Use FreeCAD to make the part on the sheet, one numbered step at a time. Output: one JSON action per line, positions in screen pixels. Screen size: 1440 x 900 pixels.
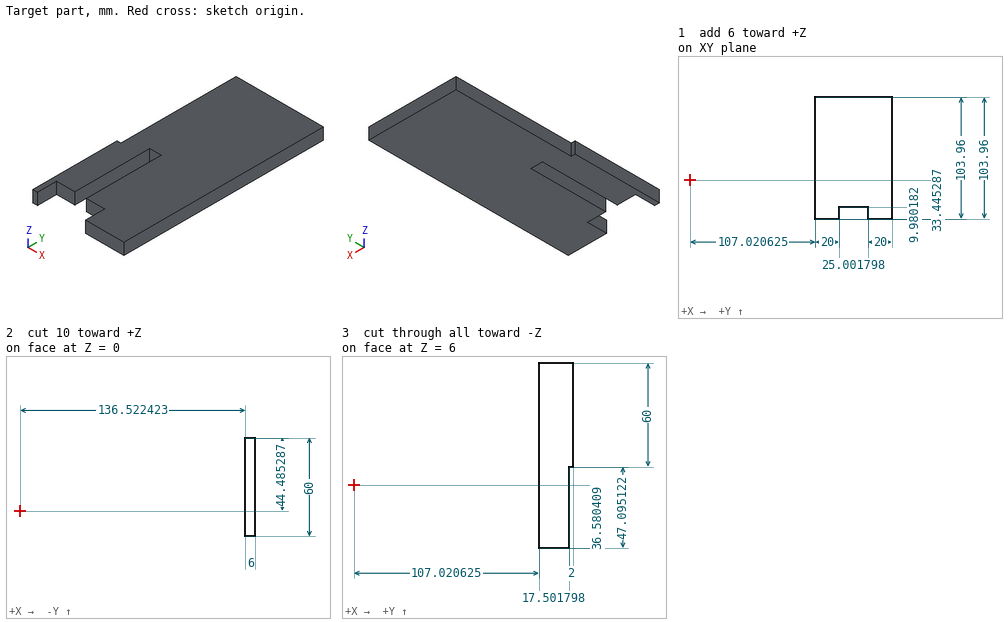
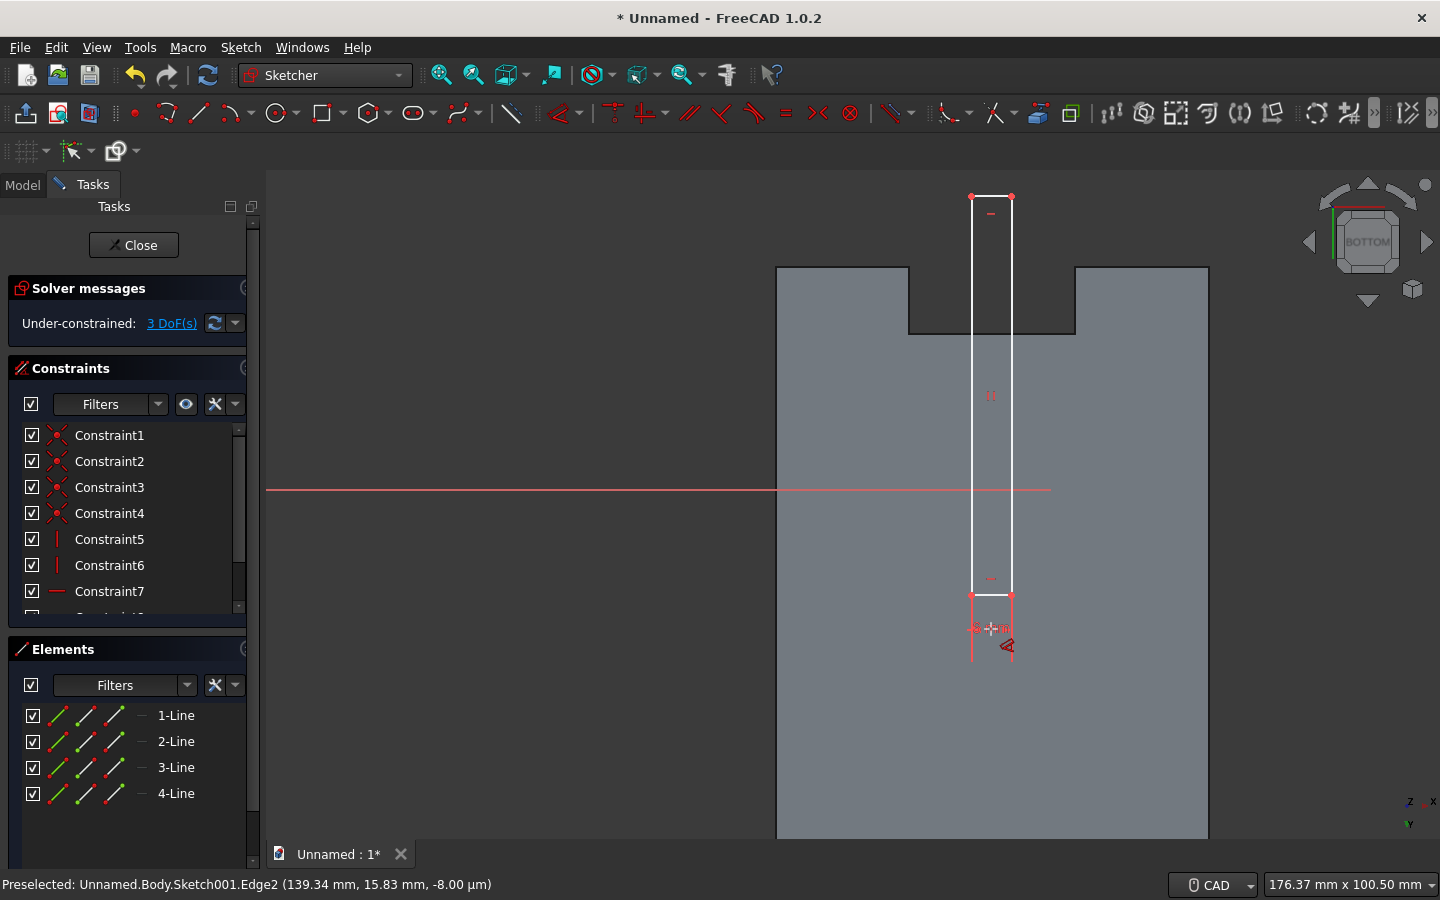
{"action": "left_click", "coordinate": [972, 316]}
{"action": "left_click", "coordinate": [938, 397]}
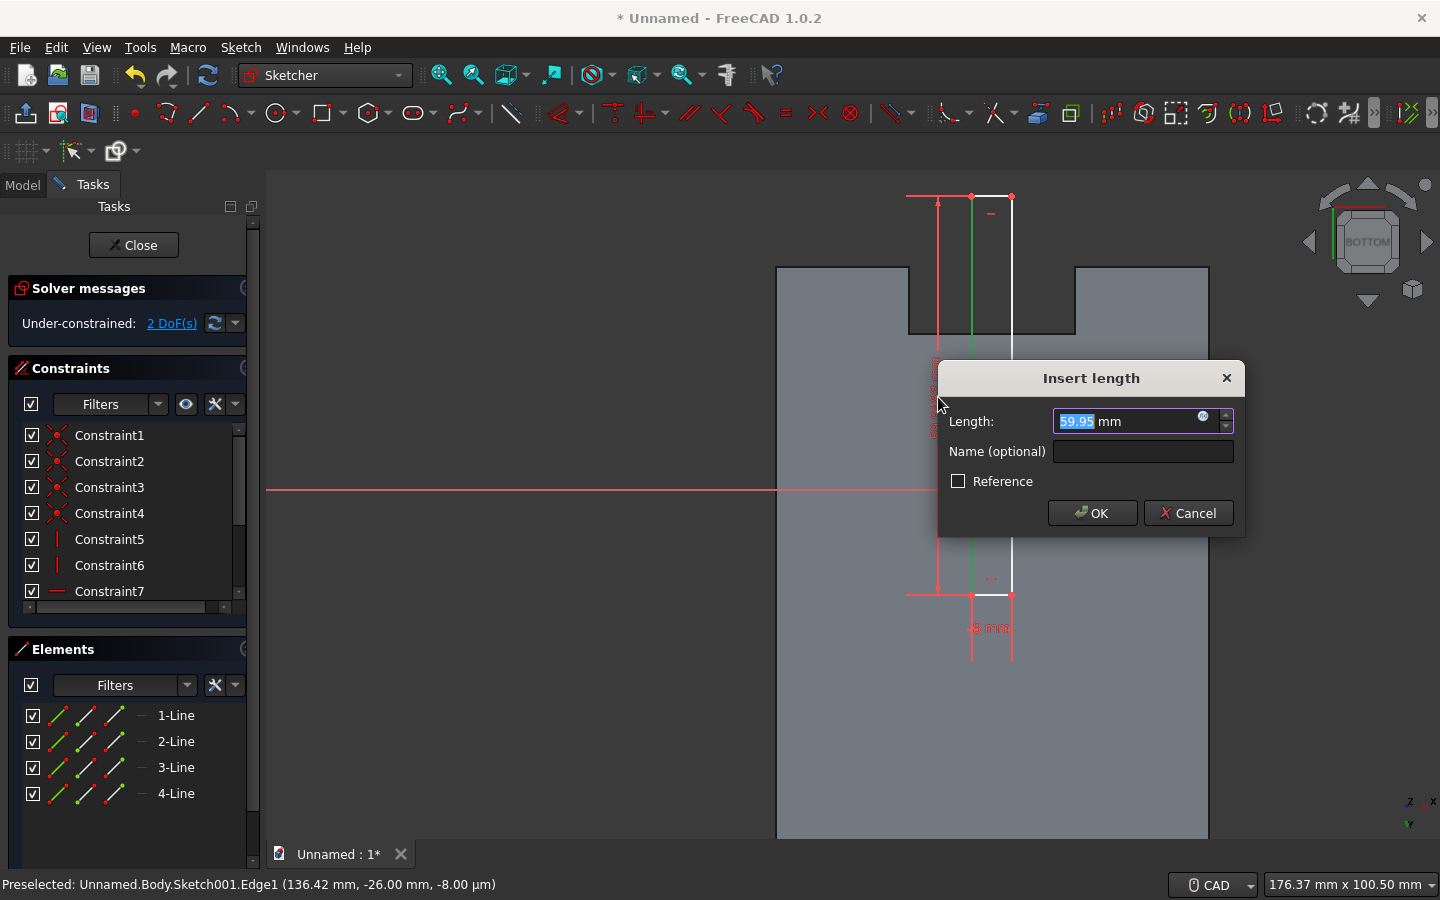
{"action": "type", "text": "60"}
{"action": "key", "text": "Return"}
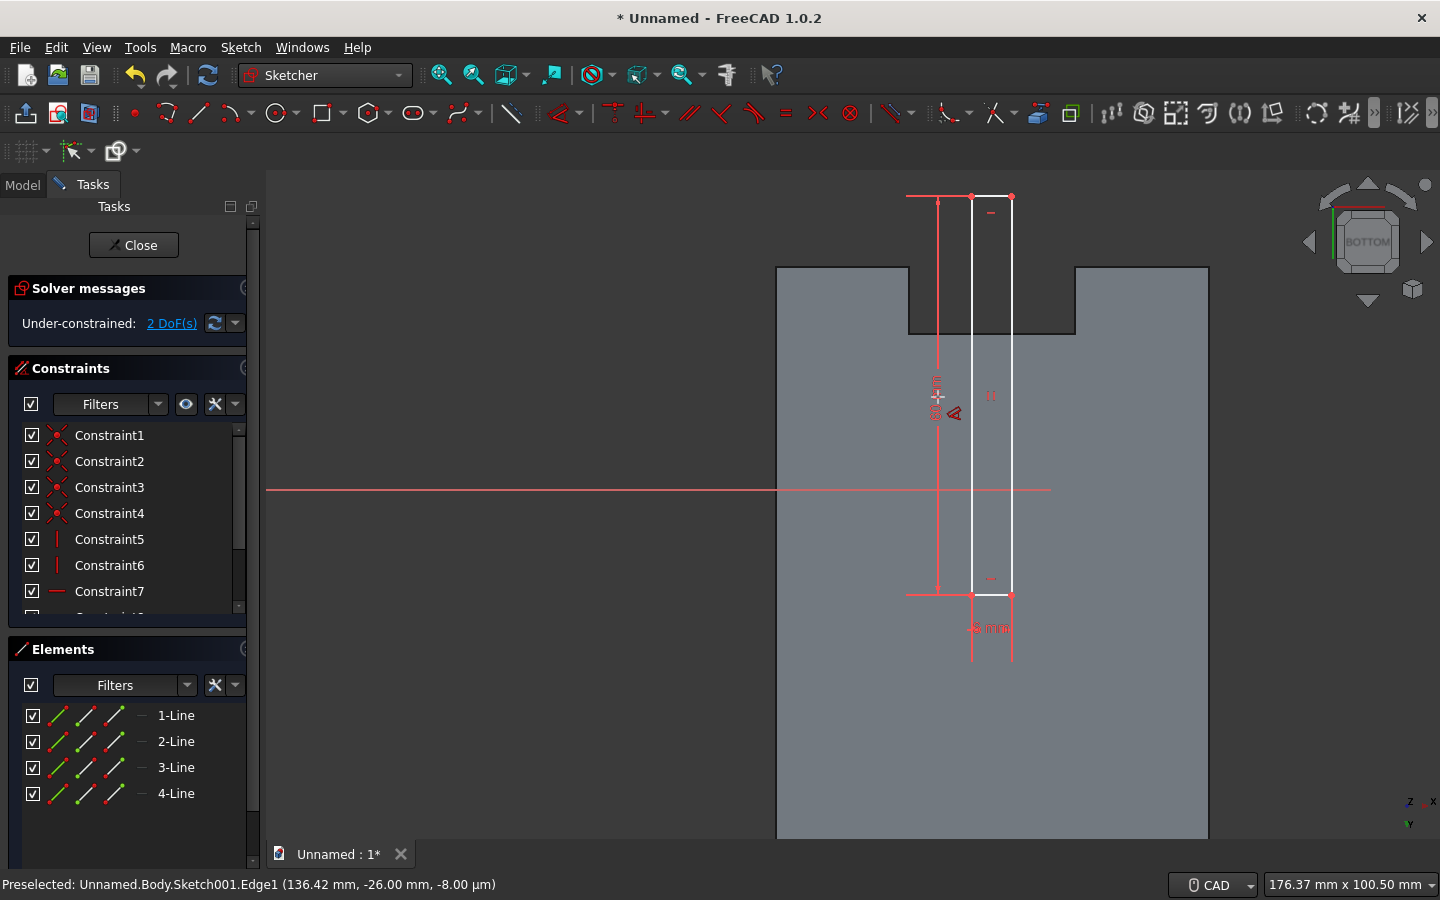
{"action": "scroll", "coordinate": [1275, 730], "scroll_direction": "down", "scroll_amount": 2}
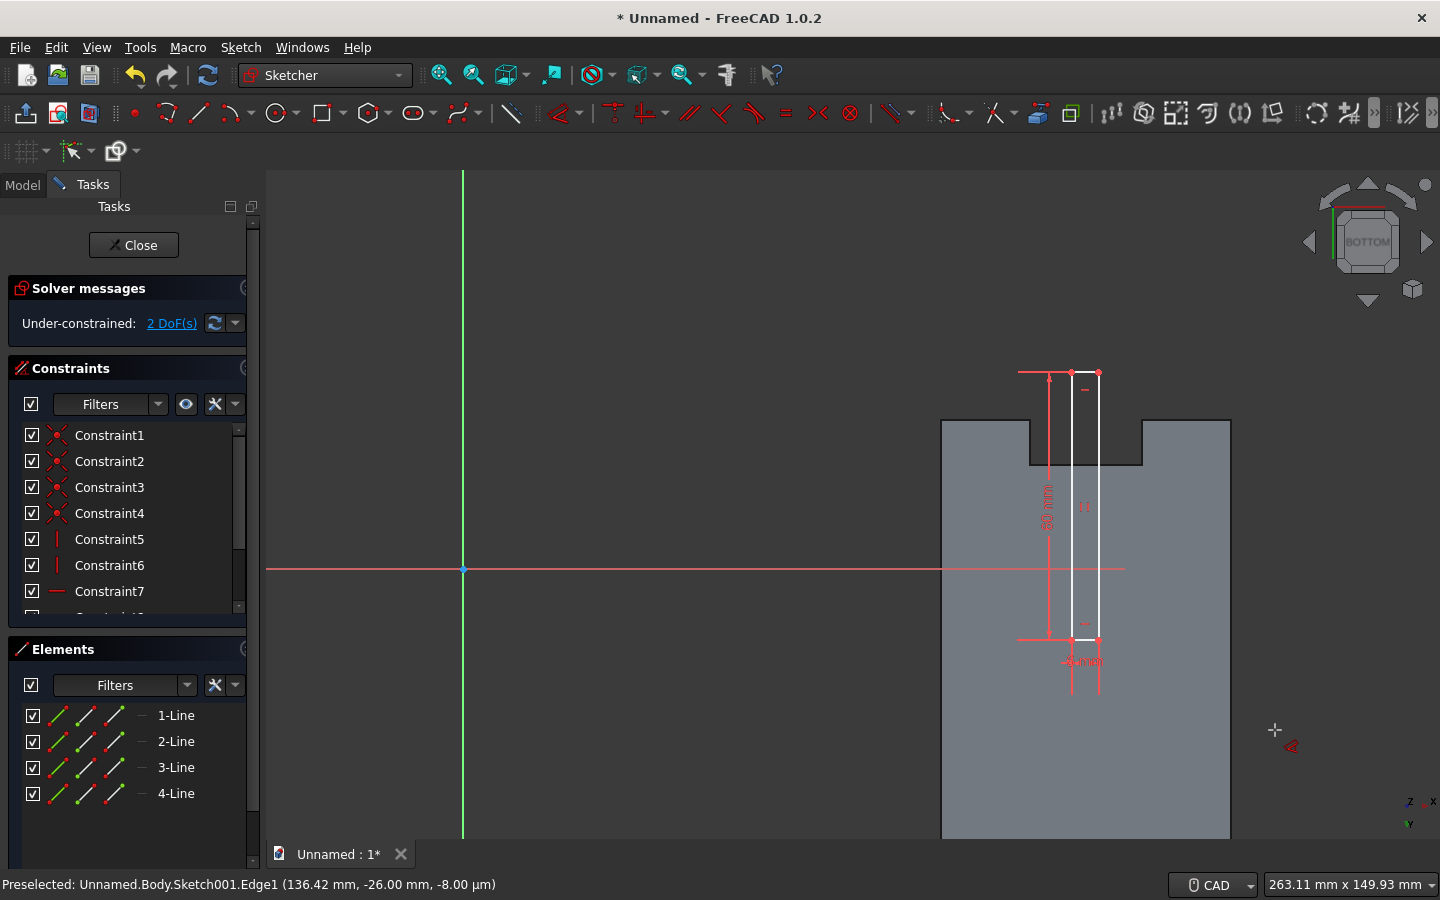
{"action": "left_click", "coordinate": [1072, 372]}
{"action": "left_click", "coordinate": [429, 471]}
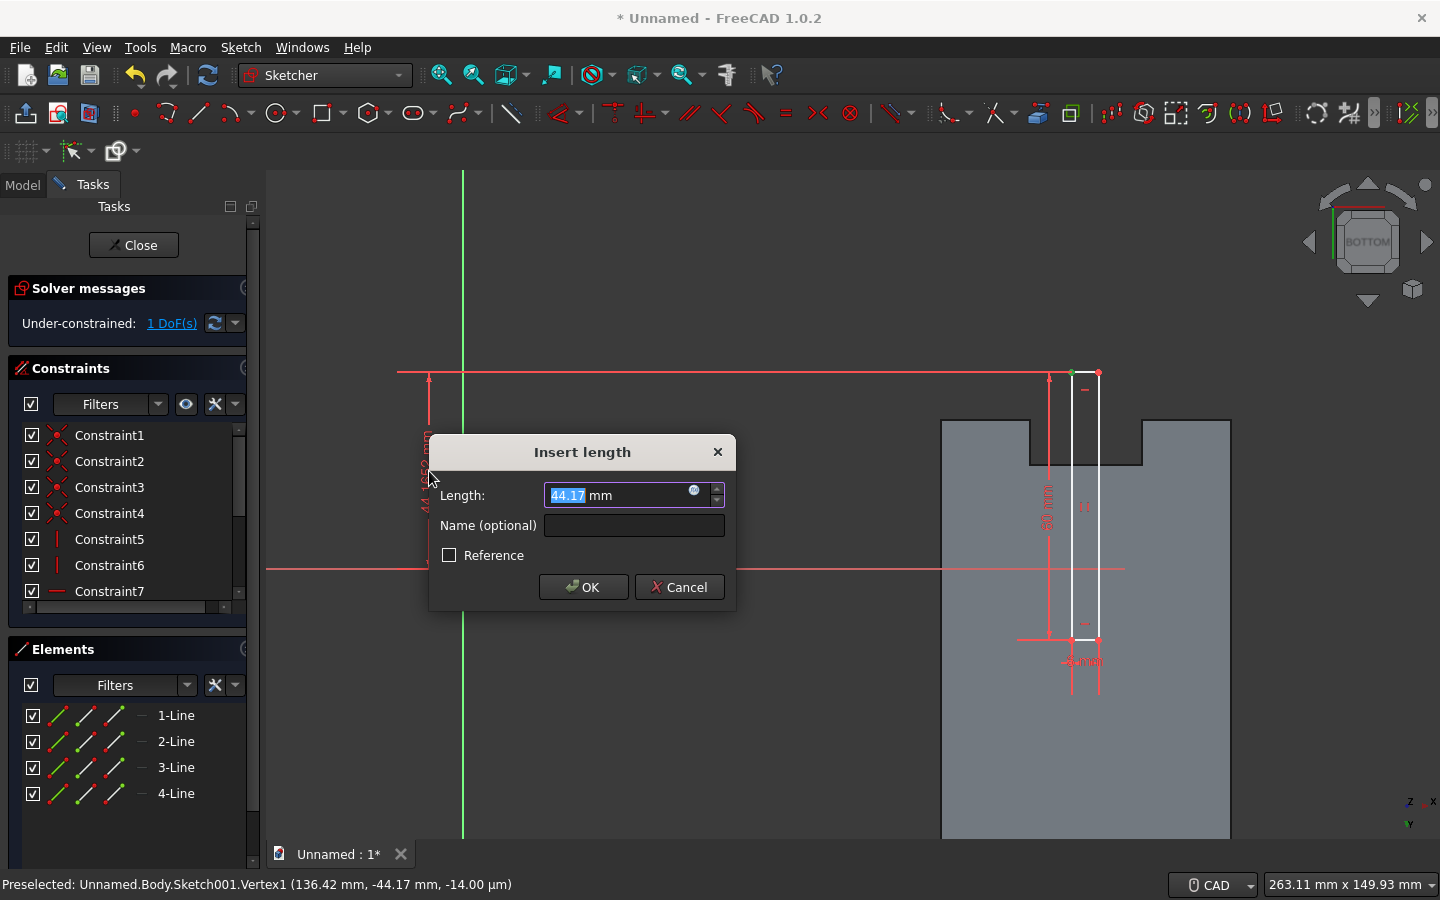
{"action": "type", "text": "44.485287"}
{"action": "key", "text": "Return"}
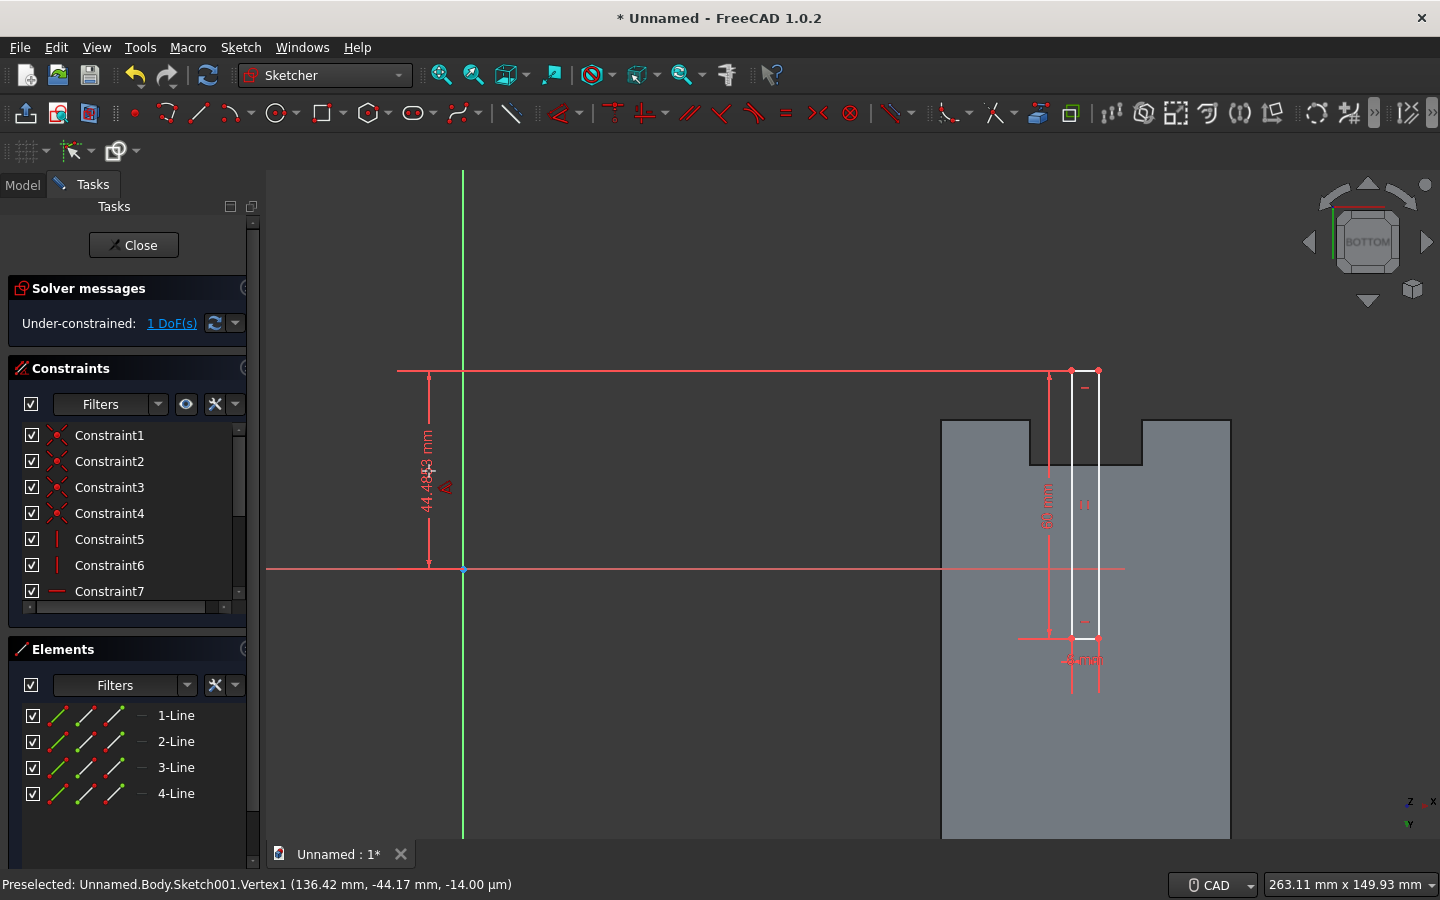
{"action": "left_click", "coordinate": [1072, 371]}
{"action": "left_click", "coordinate": [768, 337]}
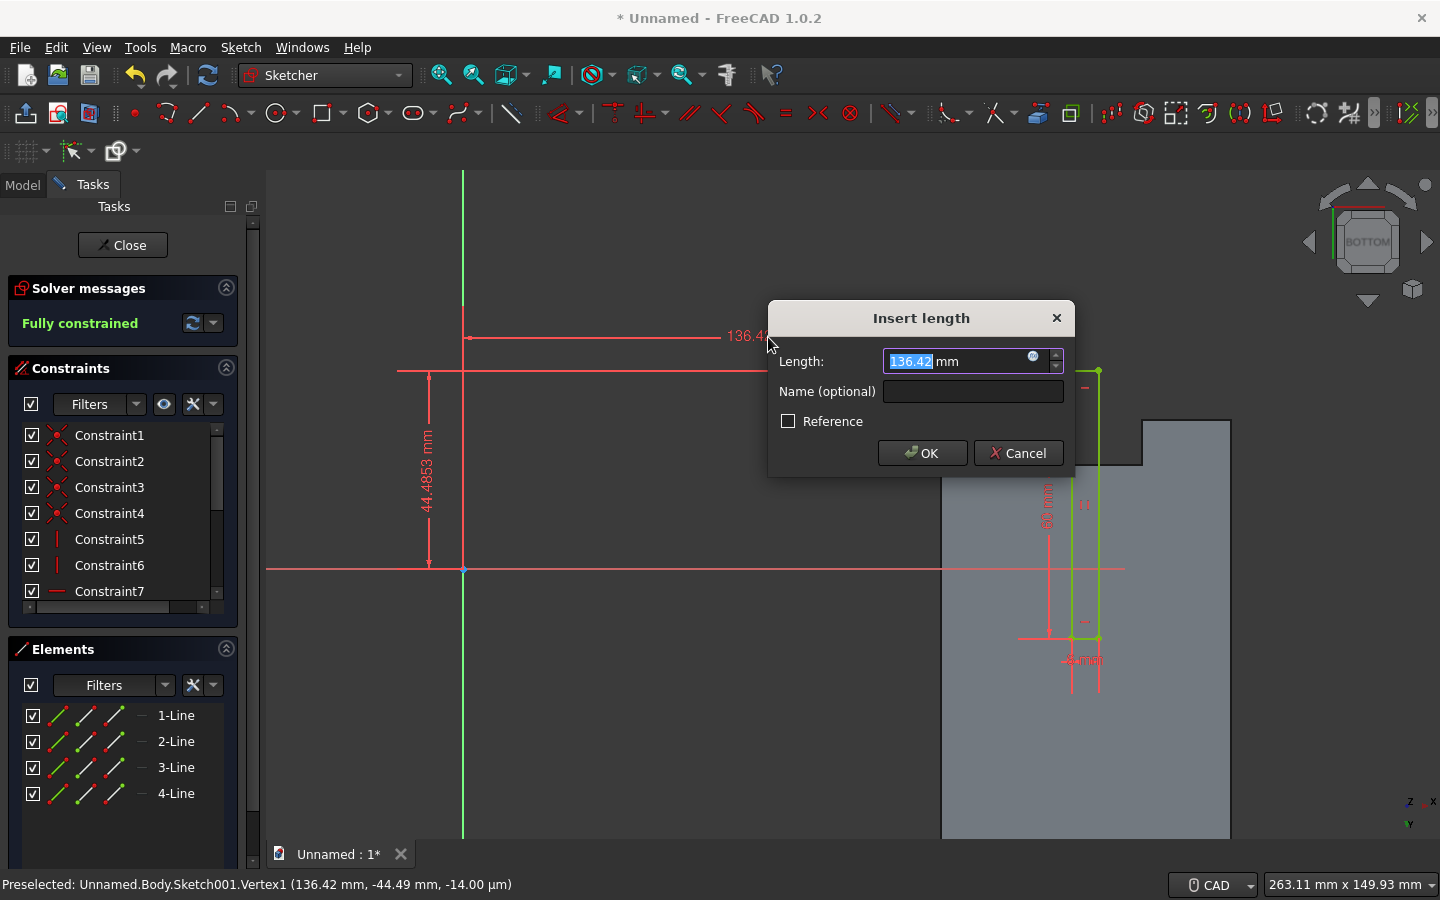
{"action": "type", "text": "136.522423"}
{"action": "key", "text": "Return"}
{"action": "key", "text": "Escape"}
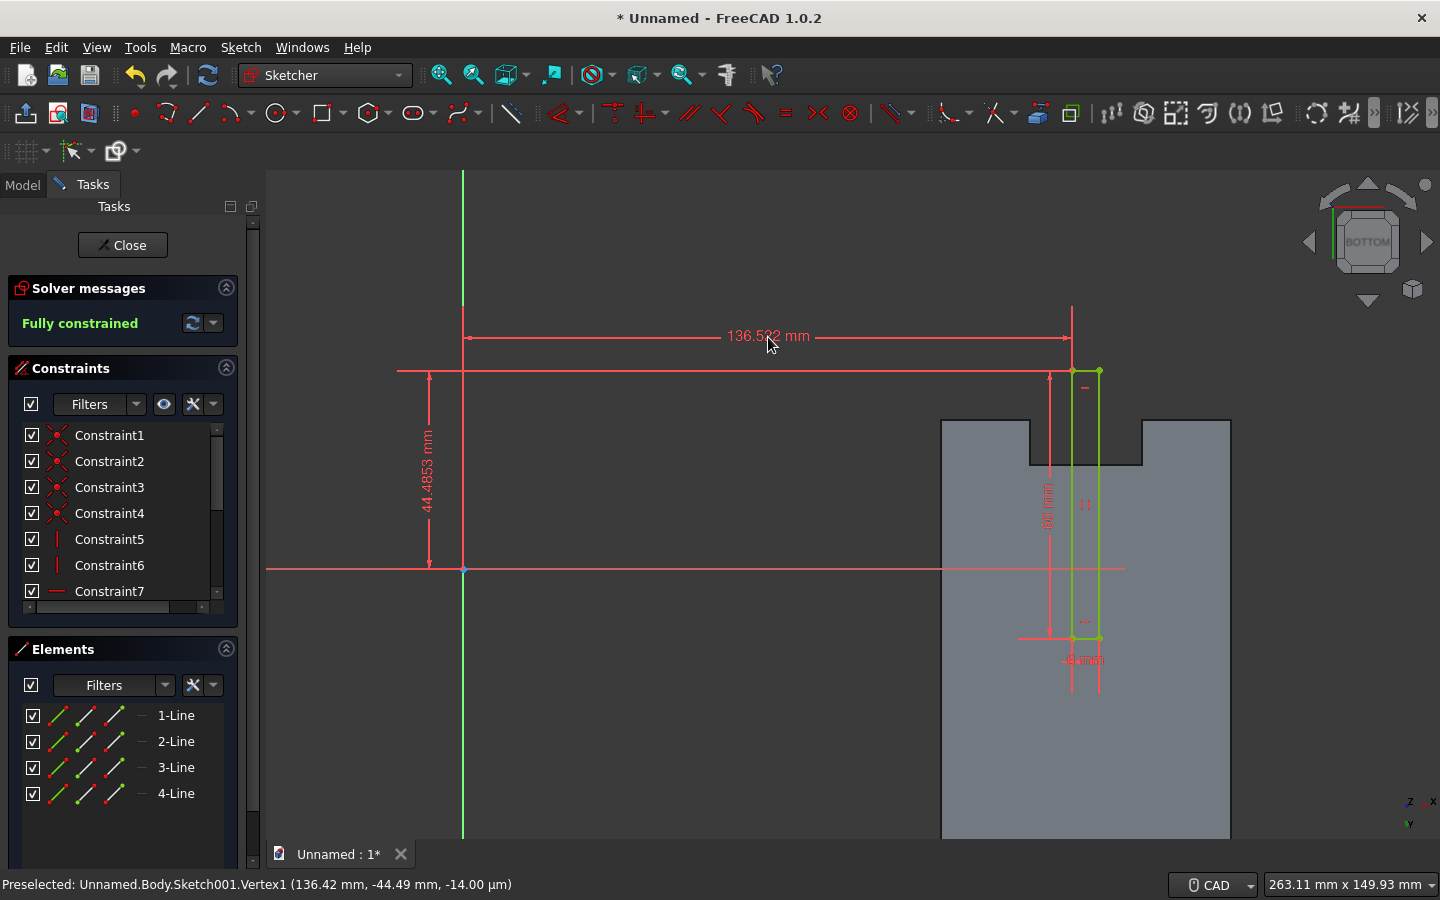
{"action": "left_click", "coordinate": [123, 245]}